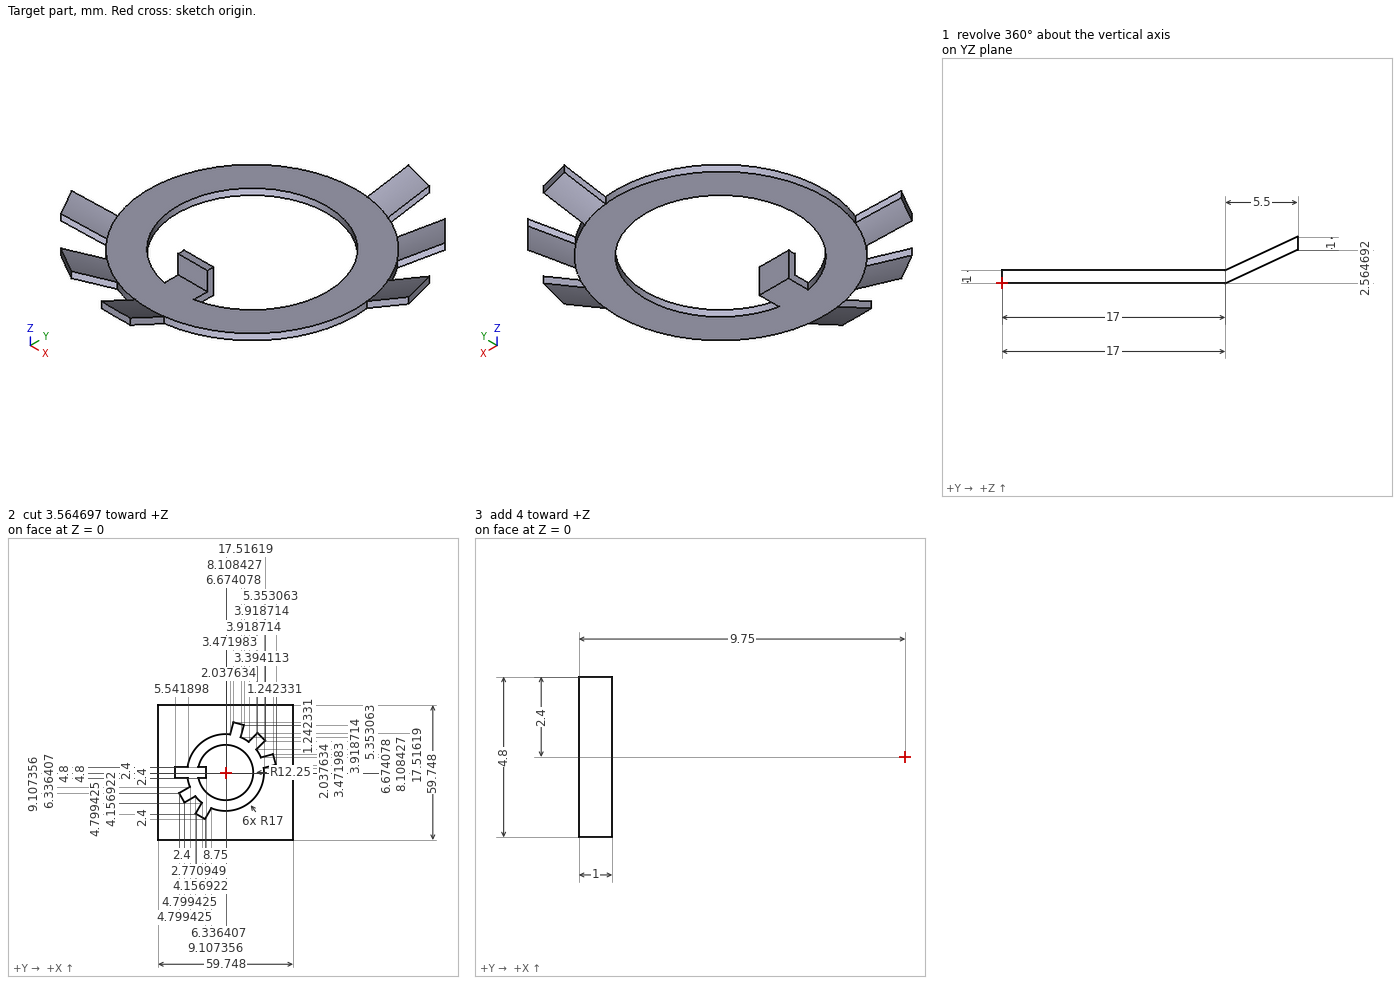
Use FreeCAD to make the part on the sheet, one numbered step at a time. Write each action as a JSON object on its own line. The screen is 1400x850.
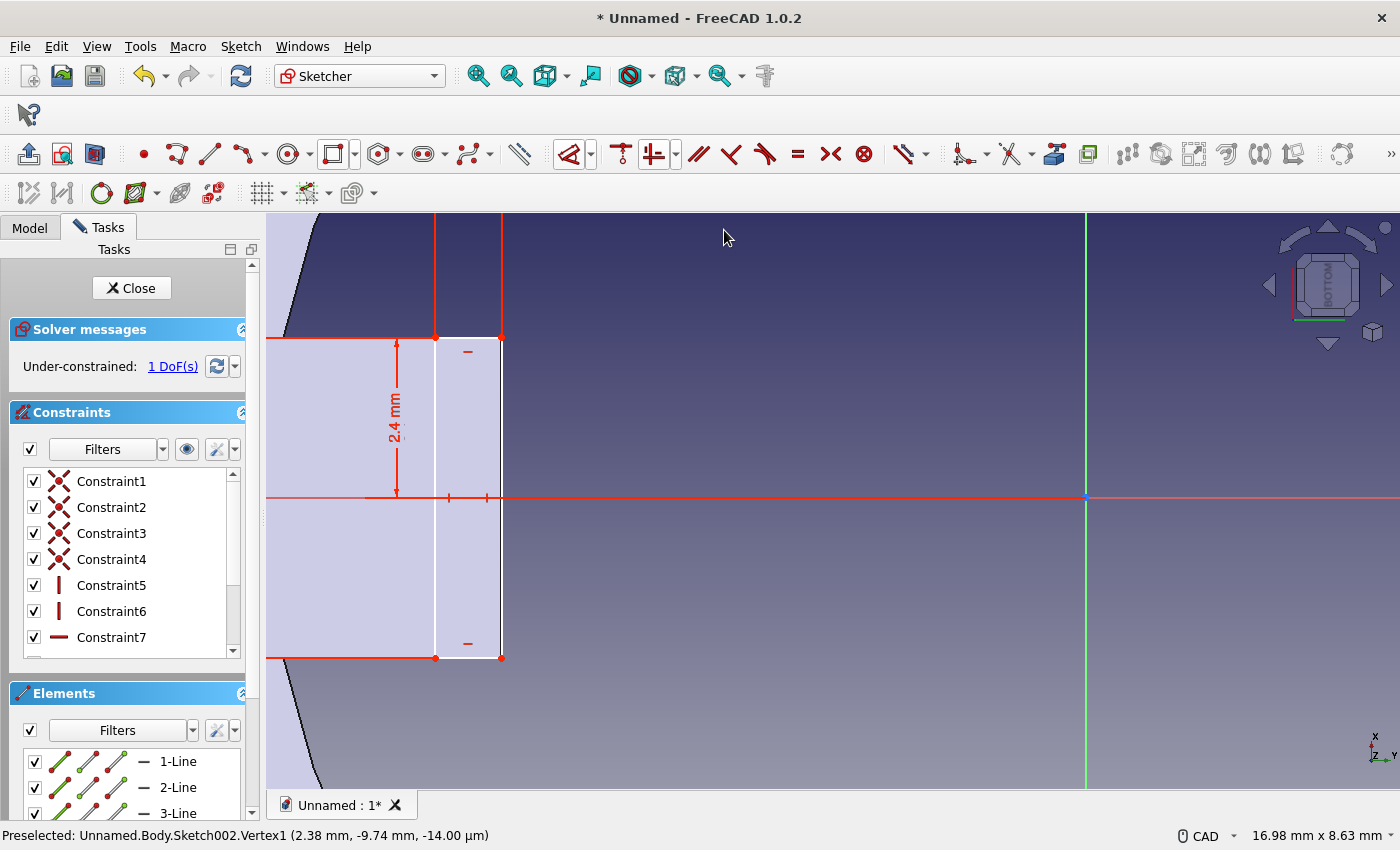
{"action": "left_click", "coordinate": [435, 338]}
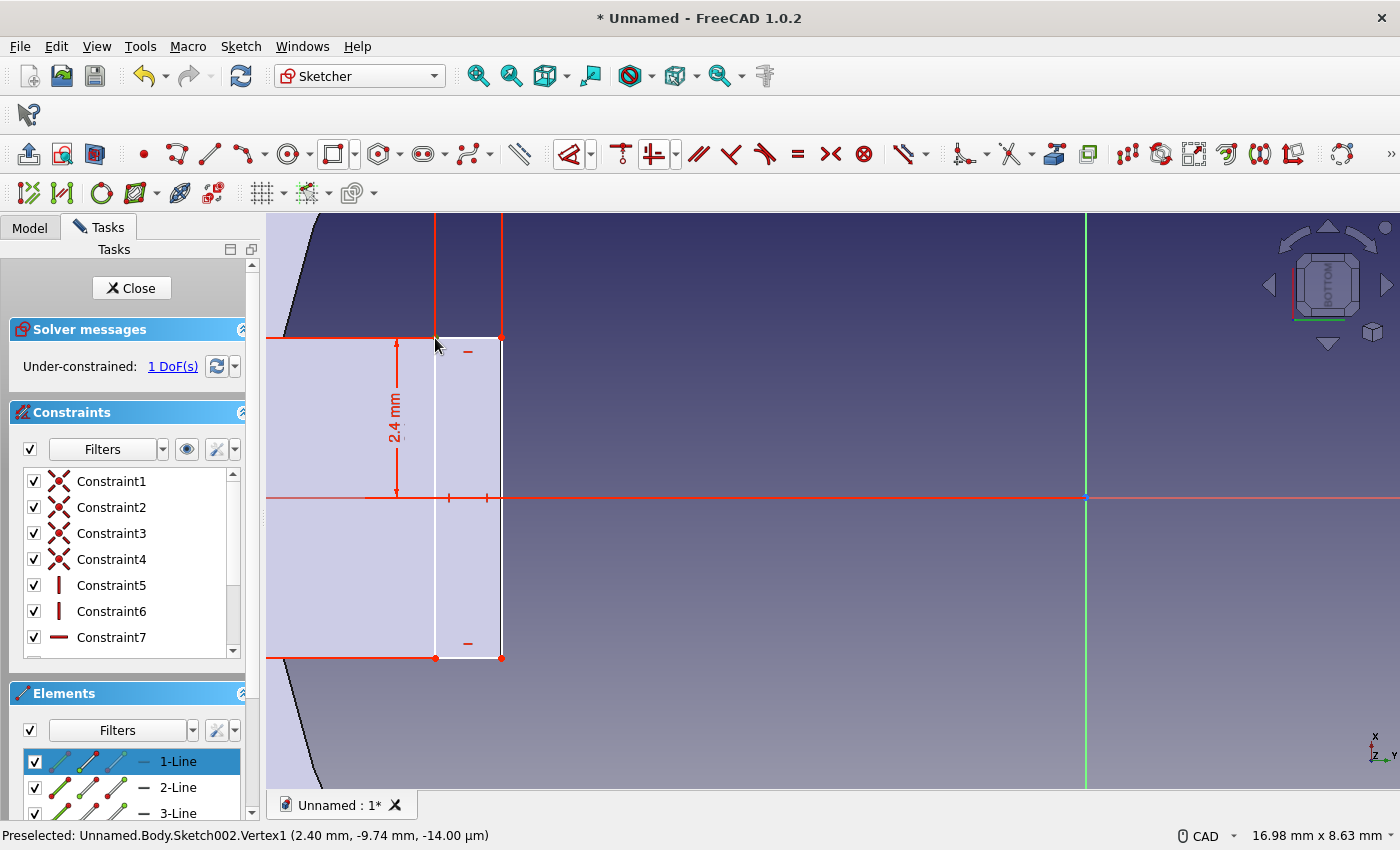
{"action": "key", "text": "l"}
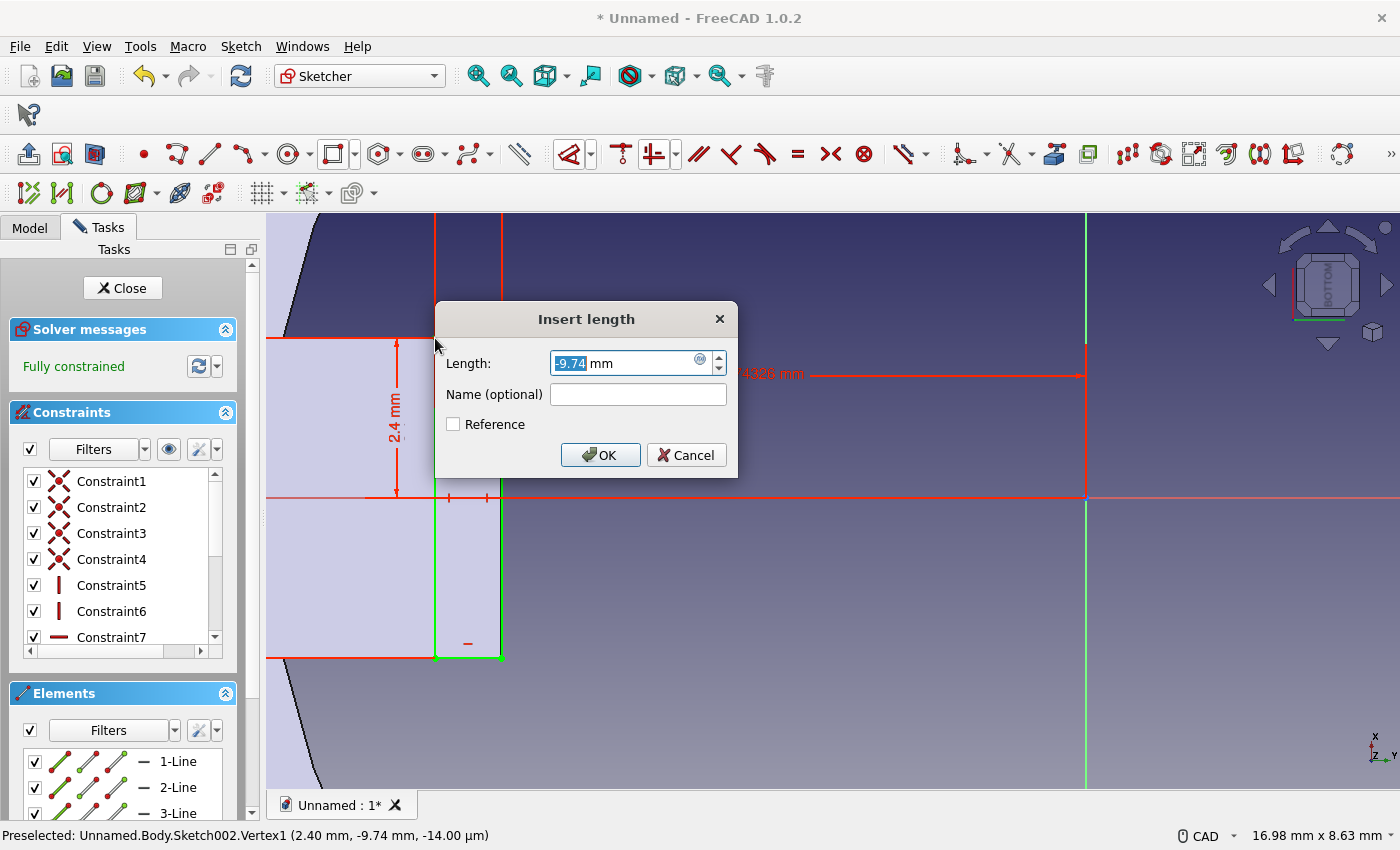
{"action": "type", "text": "-9.75"}
{"action": "key", "text": "Return"}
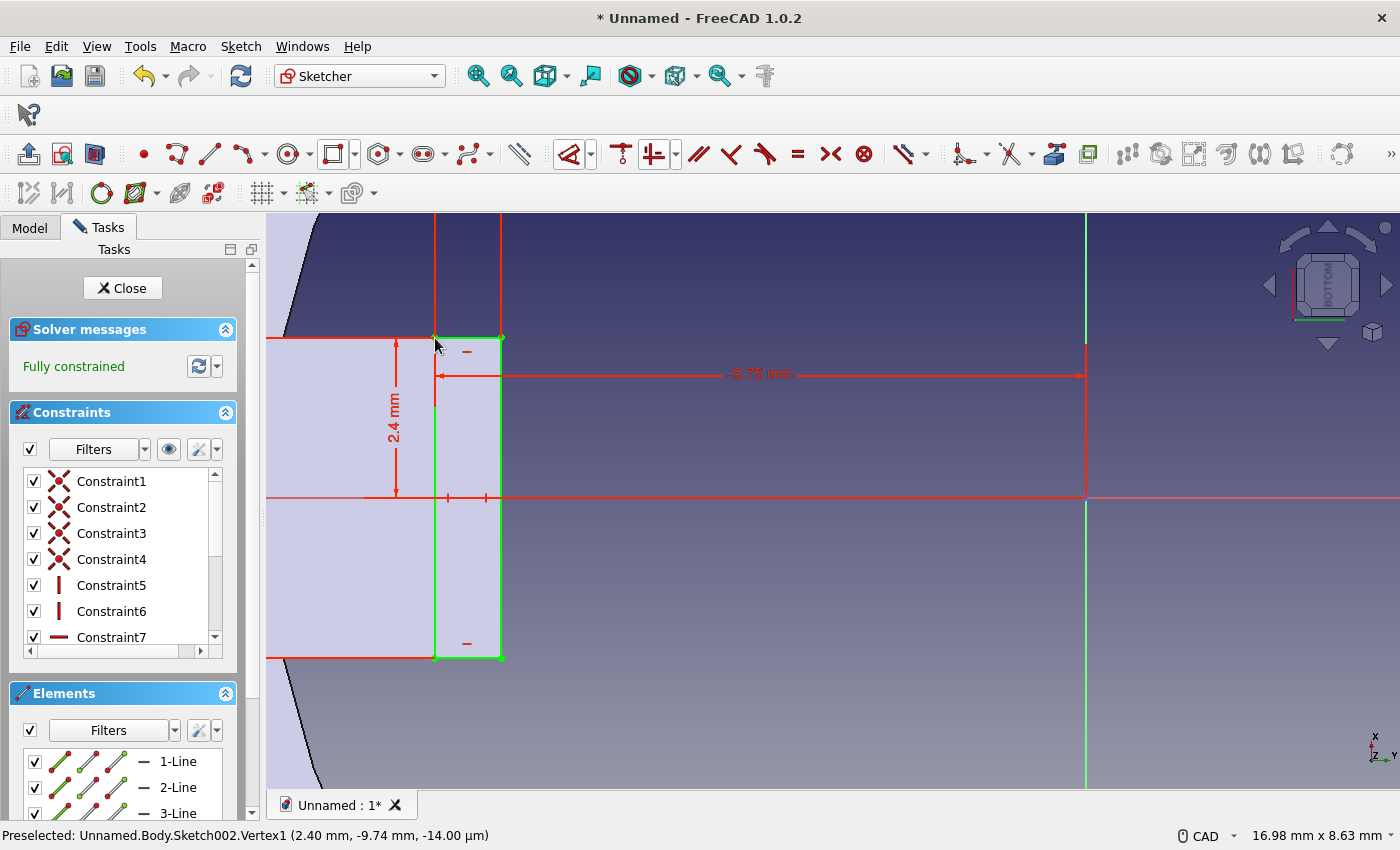
{"action": "left_click", "coordinate": [123, 288]}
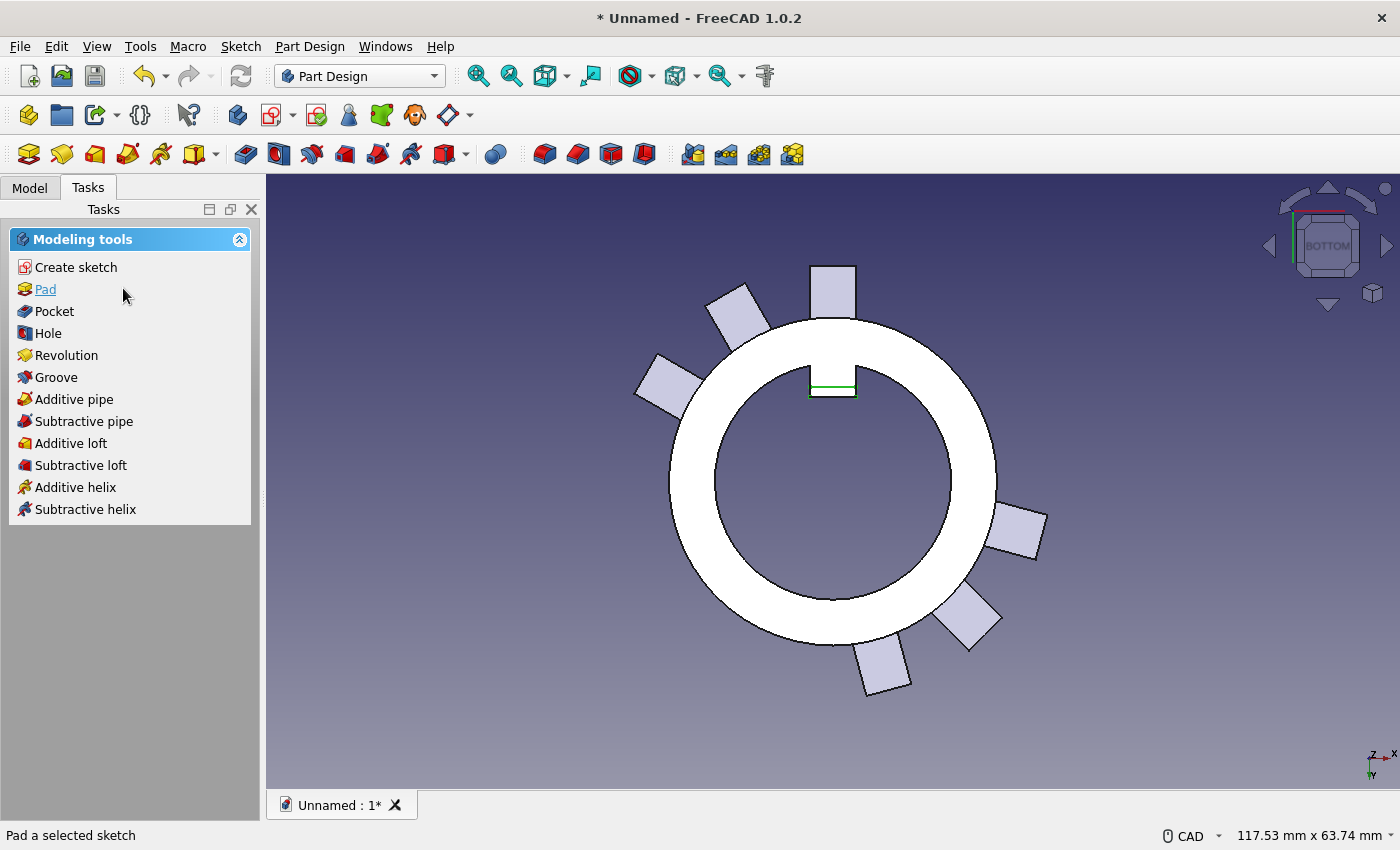
{"action": "left_click", "coordinate": [29, 154]}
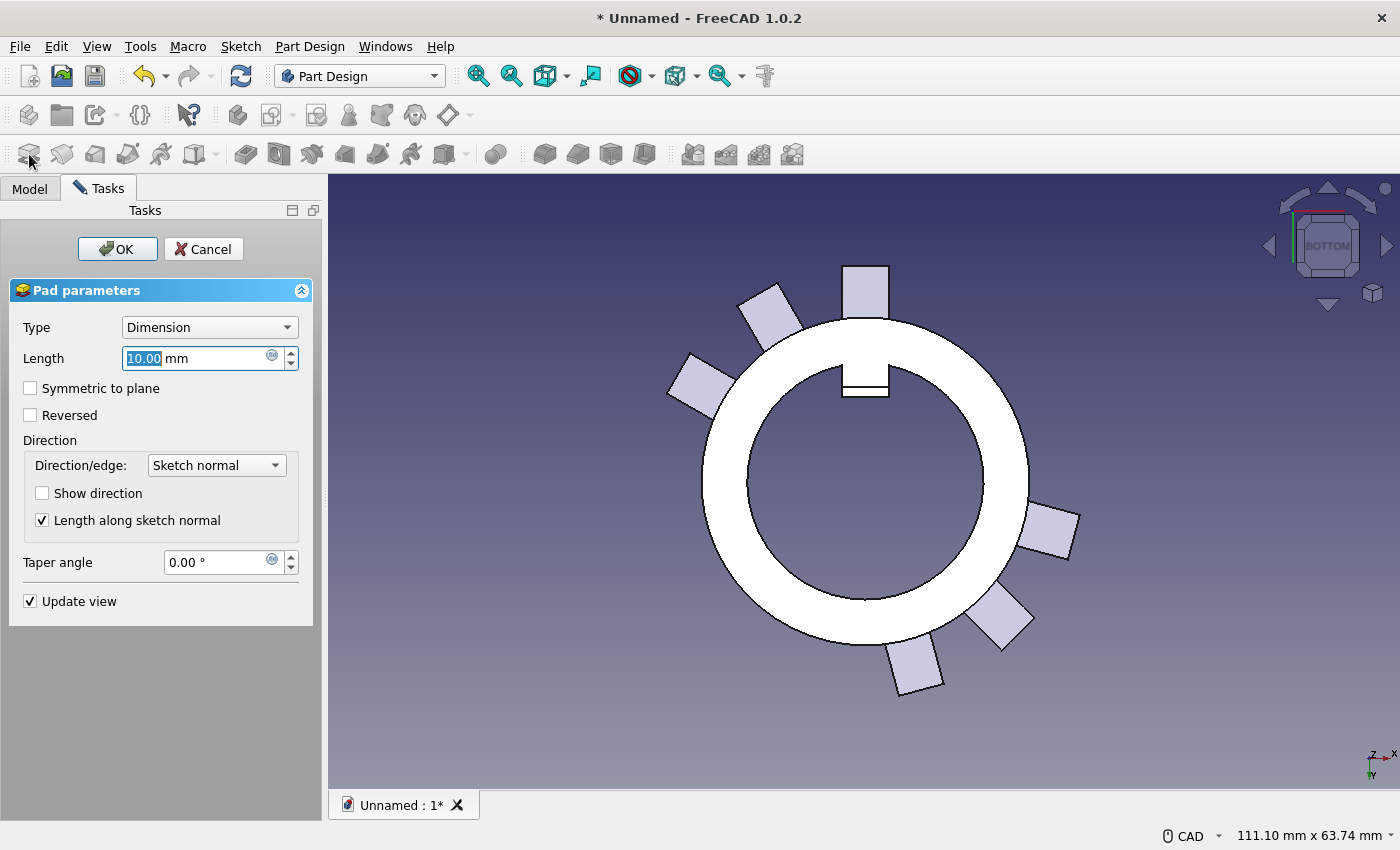
{"action": "type", "text": "4"}
{"action": "key", "text": "Tab"}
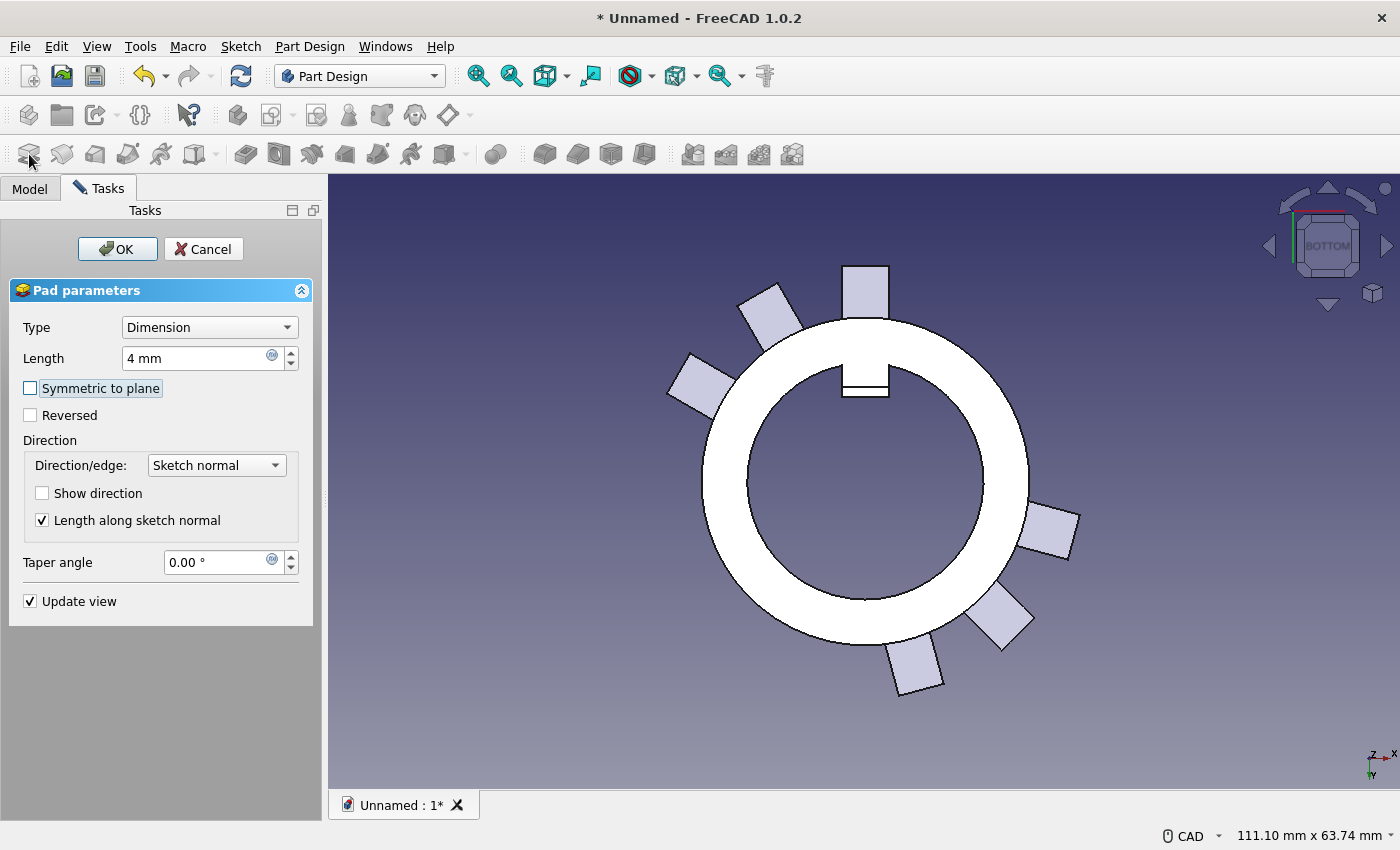
{"action": "left_click", "coordinate": [31, 415]}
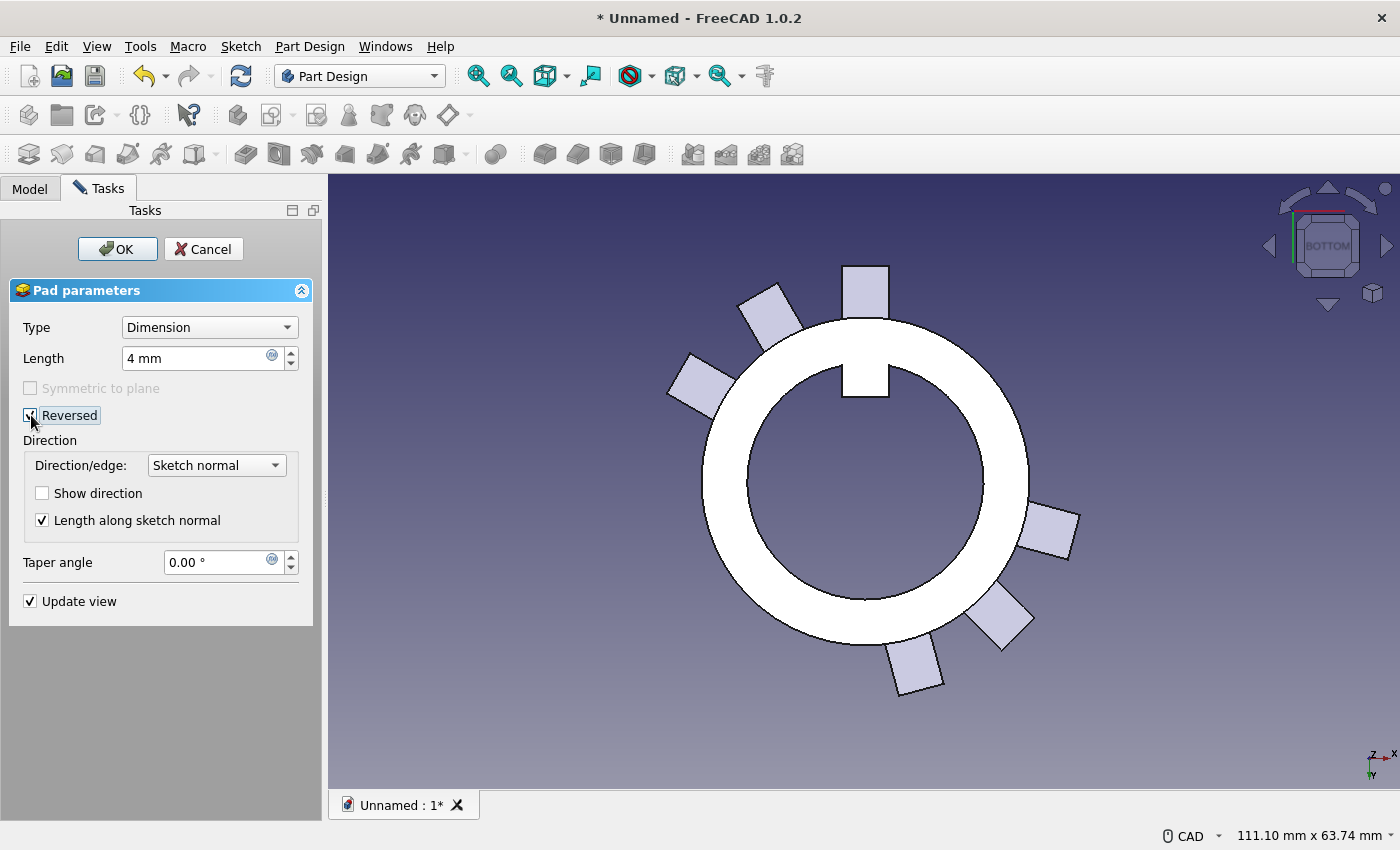
{"action": "left_click", "coordinate": [118, 249]}